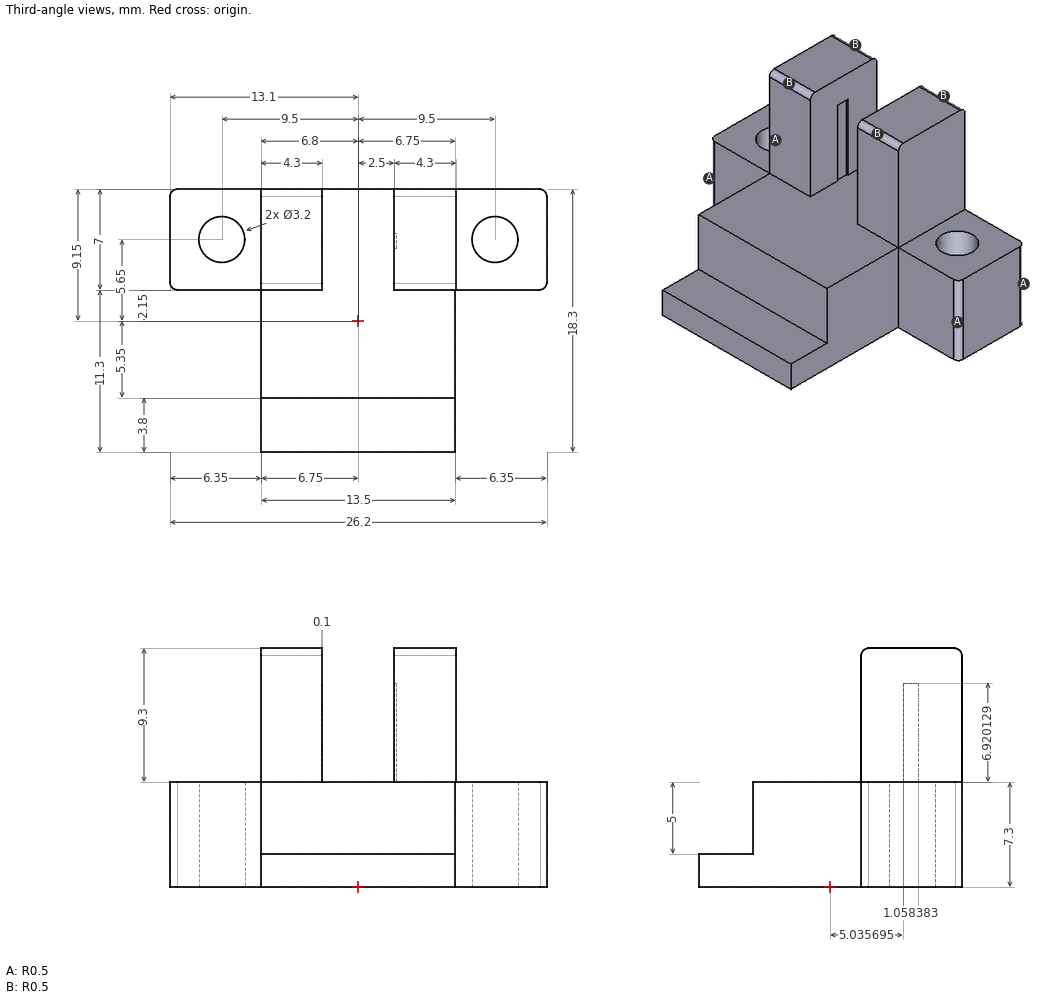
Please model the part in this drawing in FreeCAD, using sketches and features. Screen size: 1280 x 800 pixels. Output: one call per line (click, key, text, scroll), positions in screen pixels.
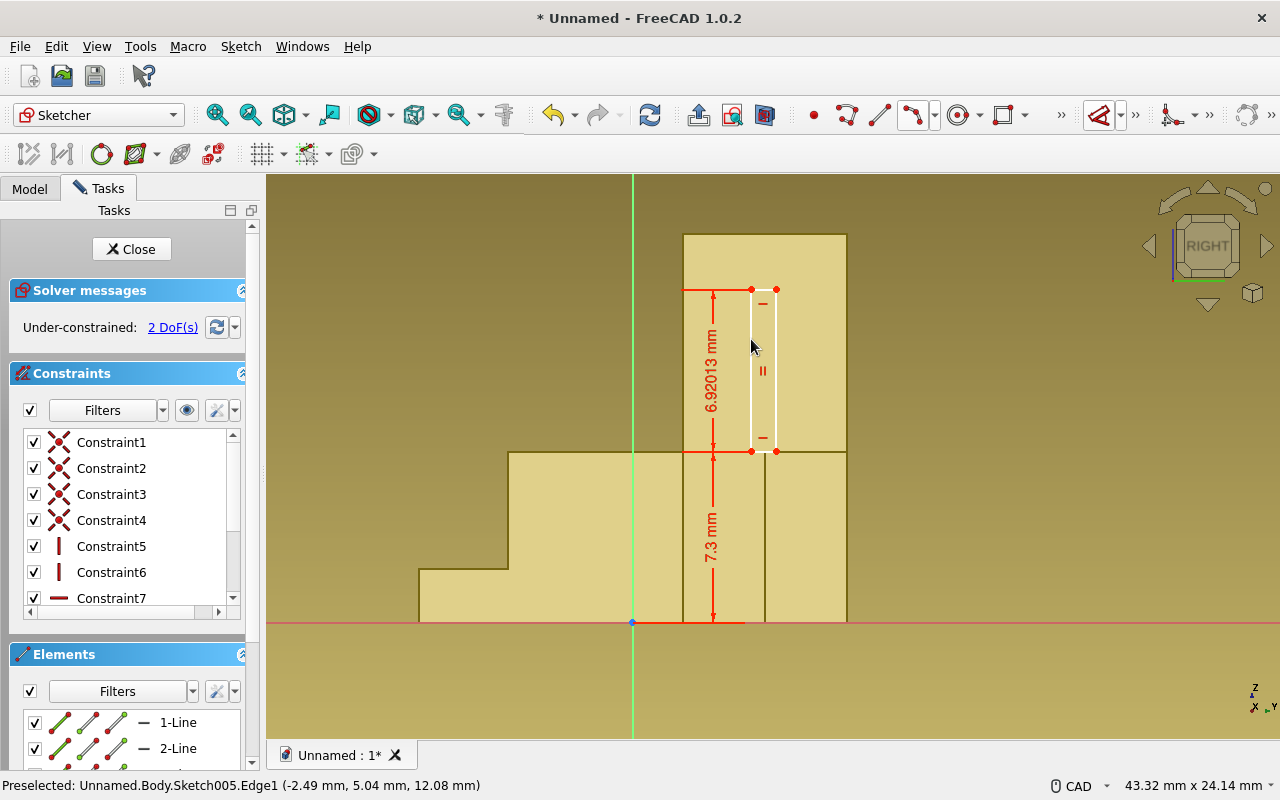
scroll(761, 452, up, 3)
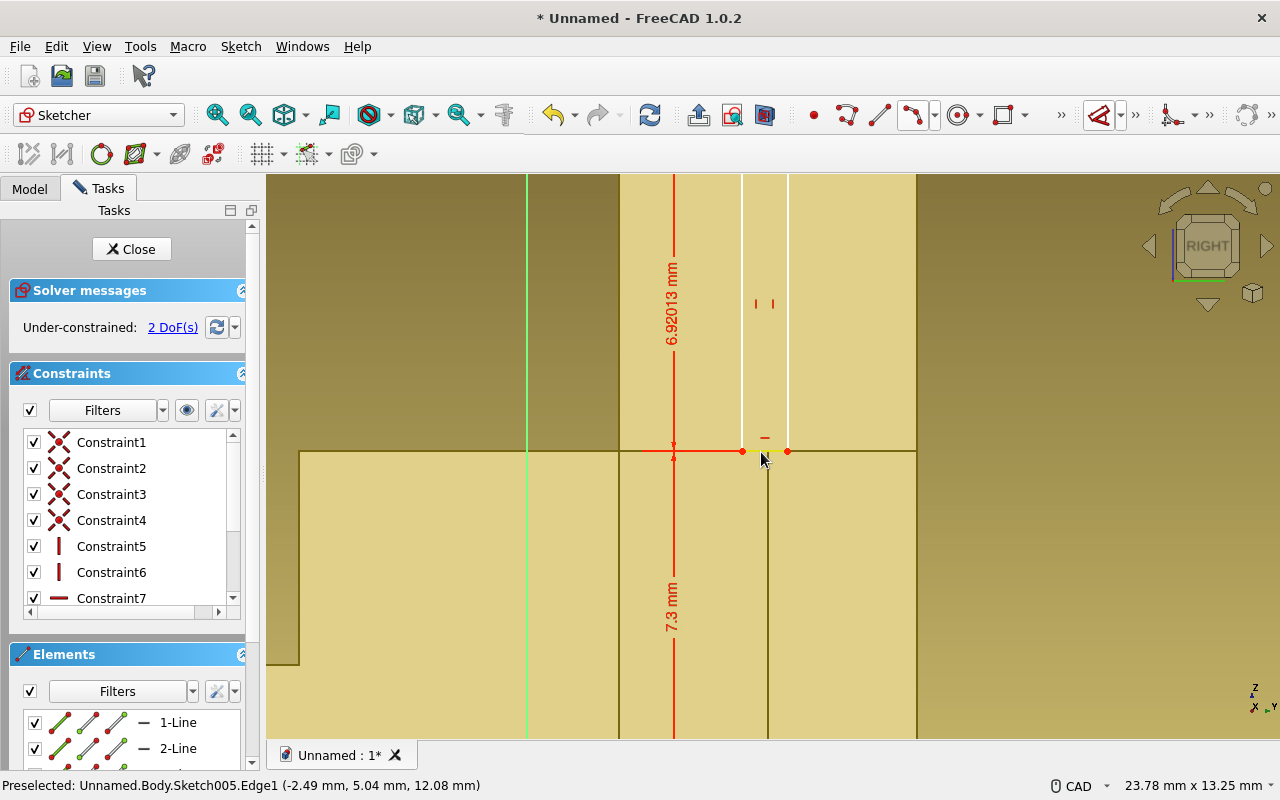
click(761, 451)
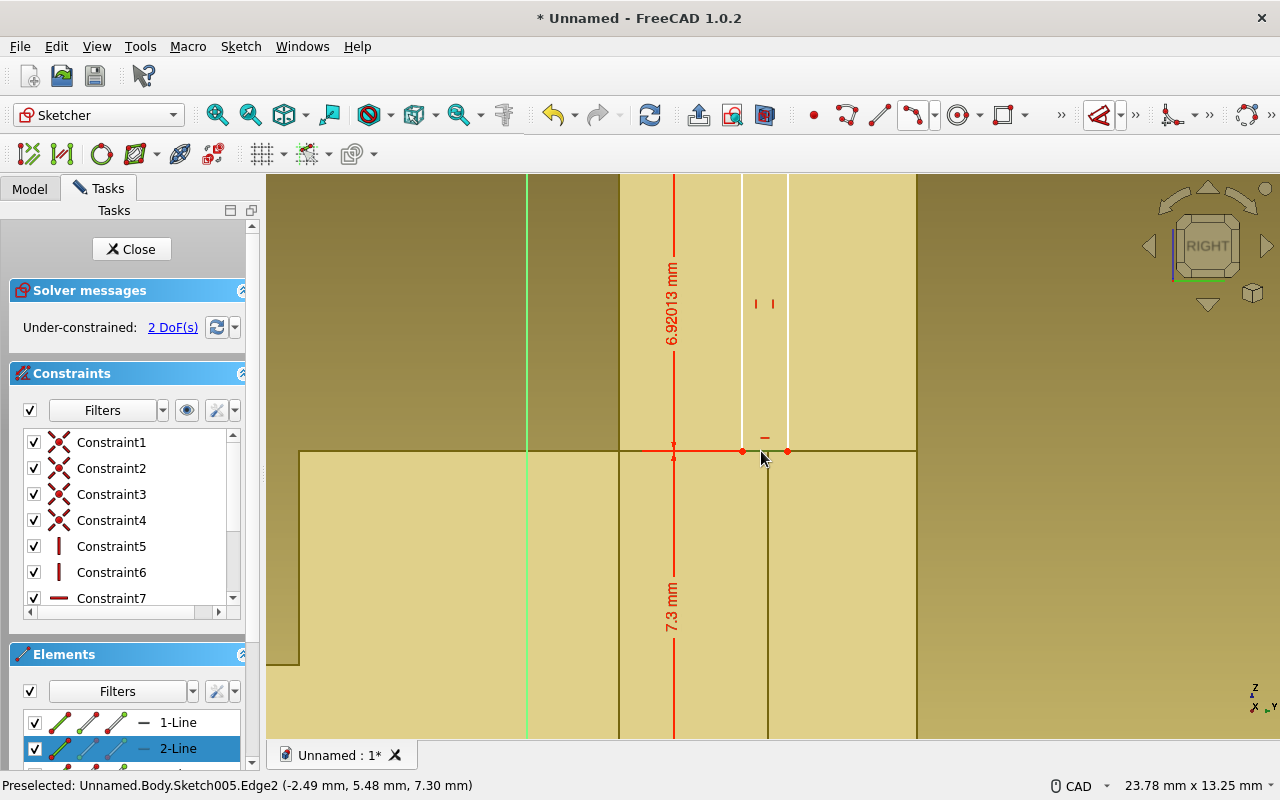
key(l)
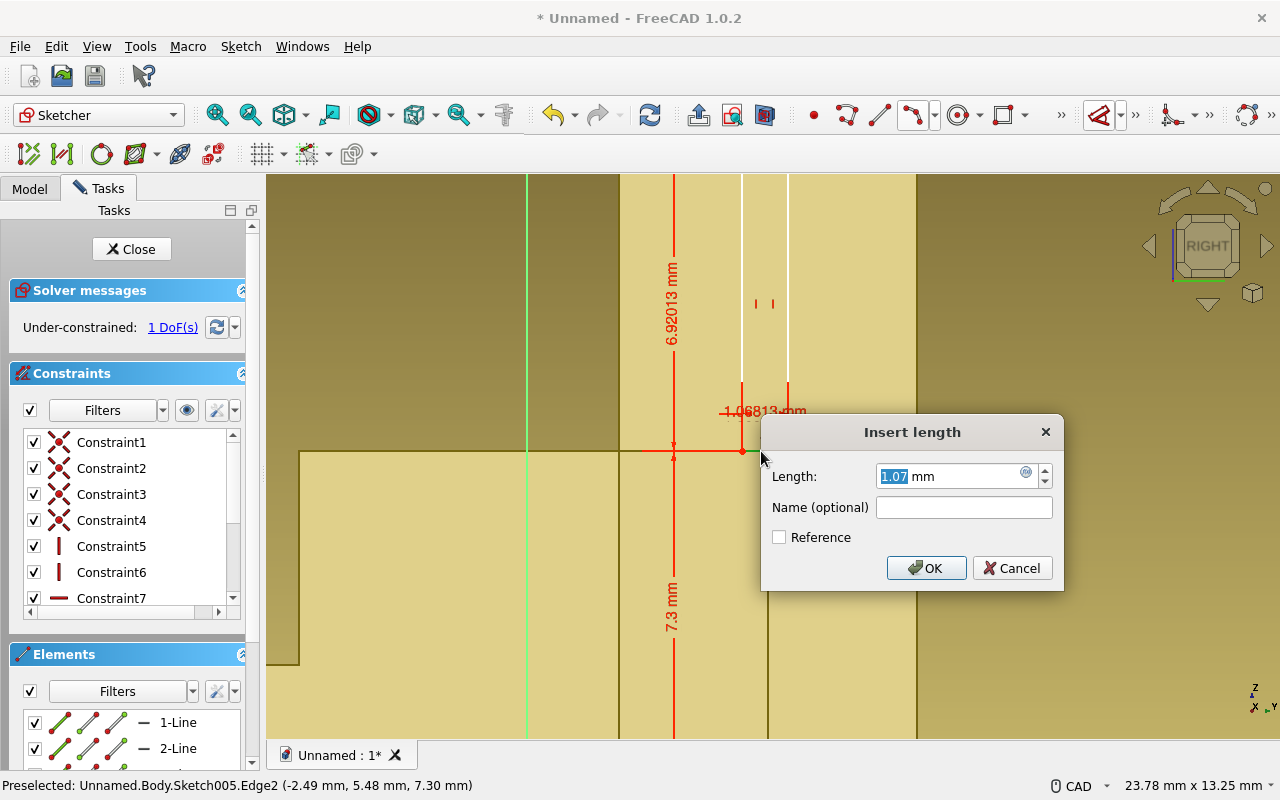
text(1.058383)
key(Return)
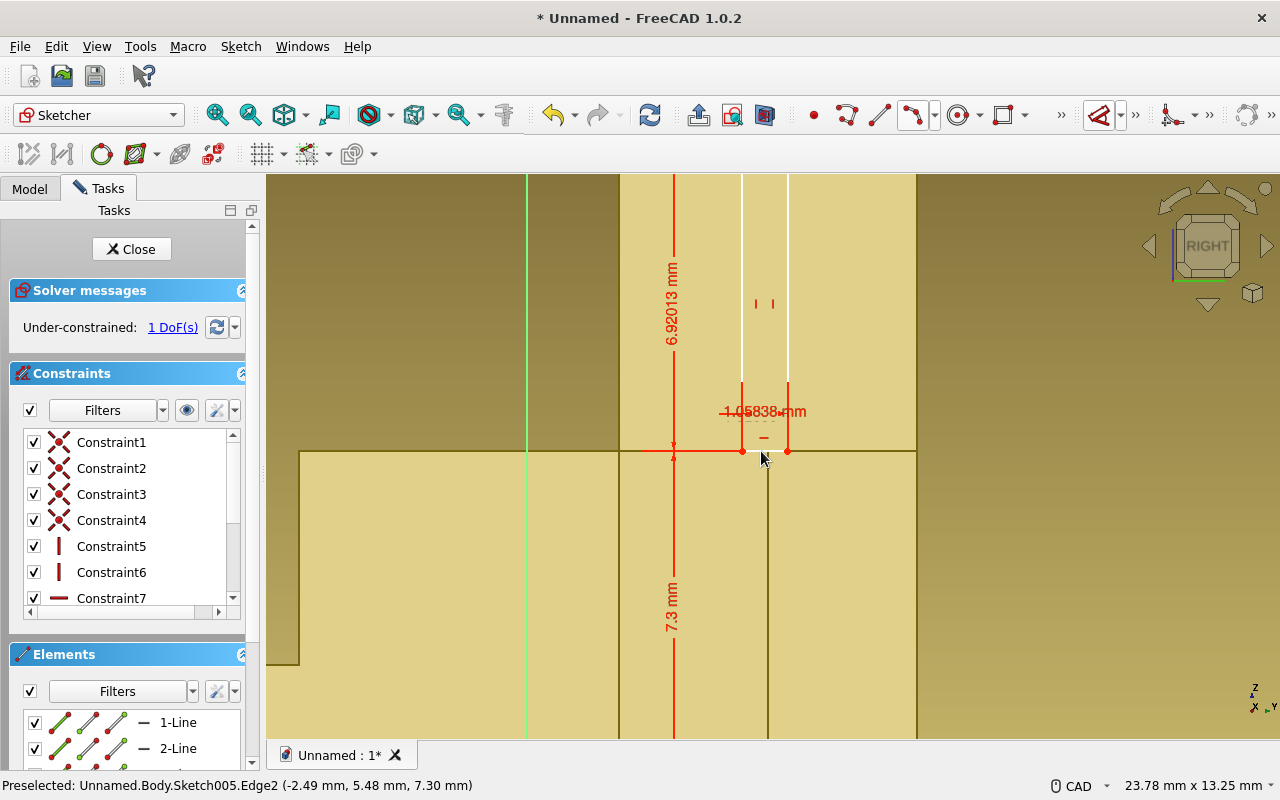
scroll(762, 453, down, 3)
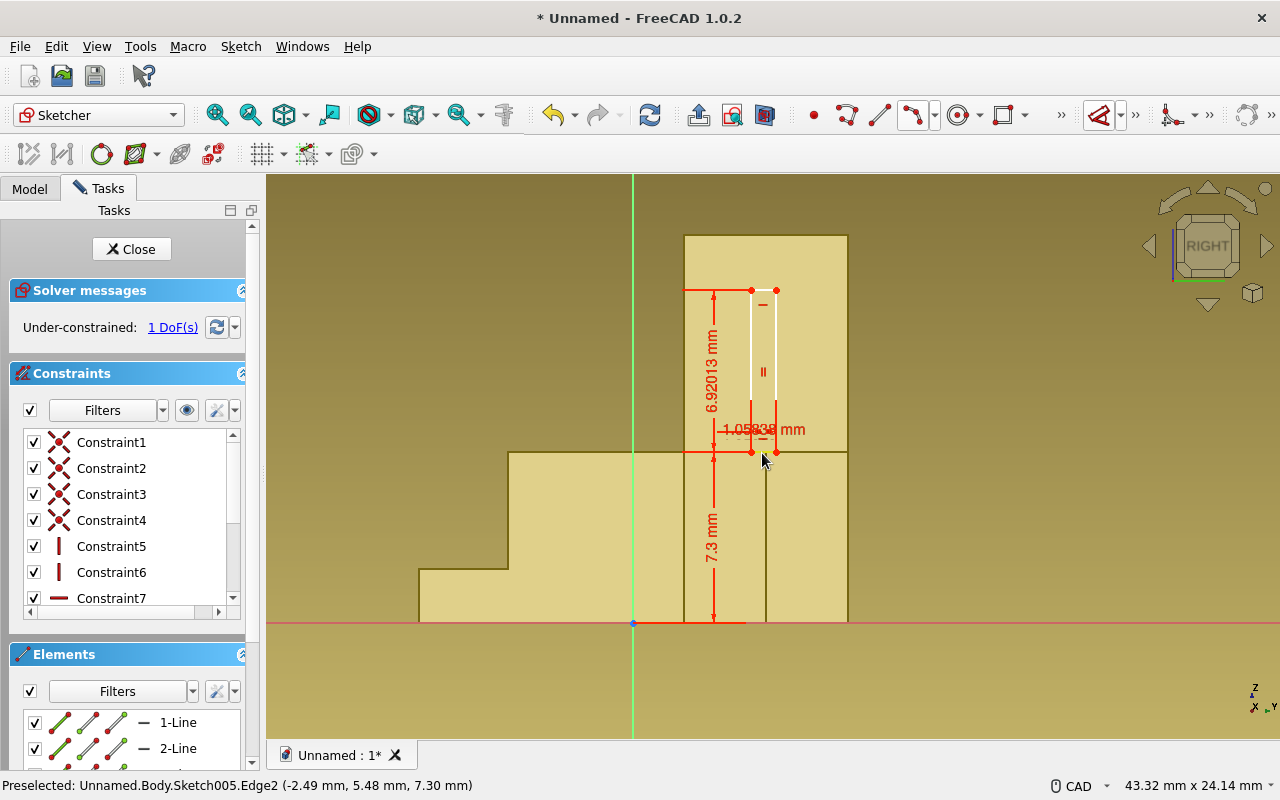
click(751, 290)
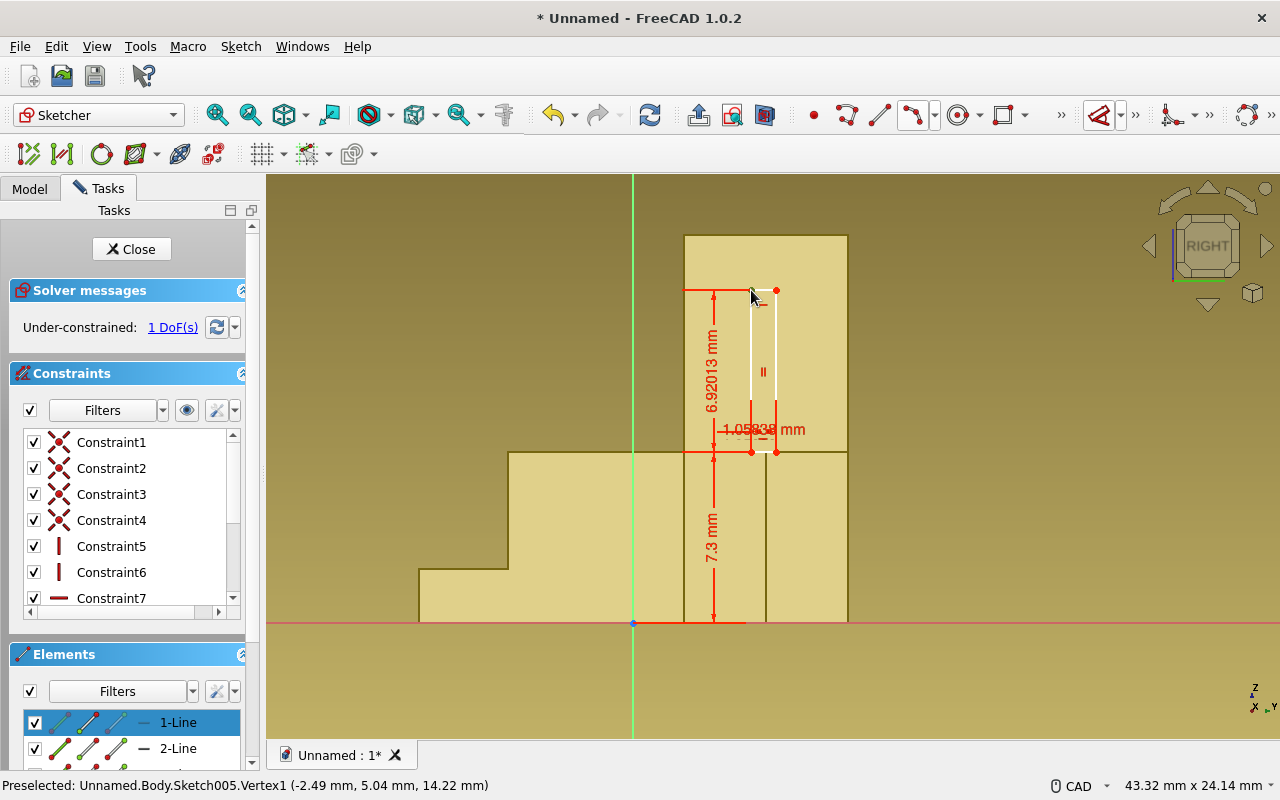
click(1120, 116)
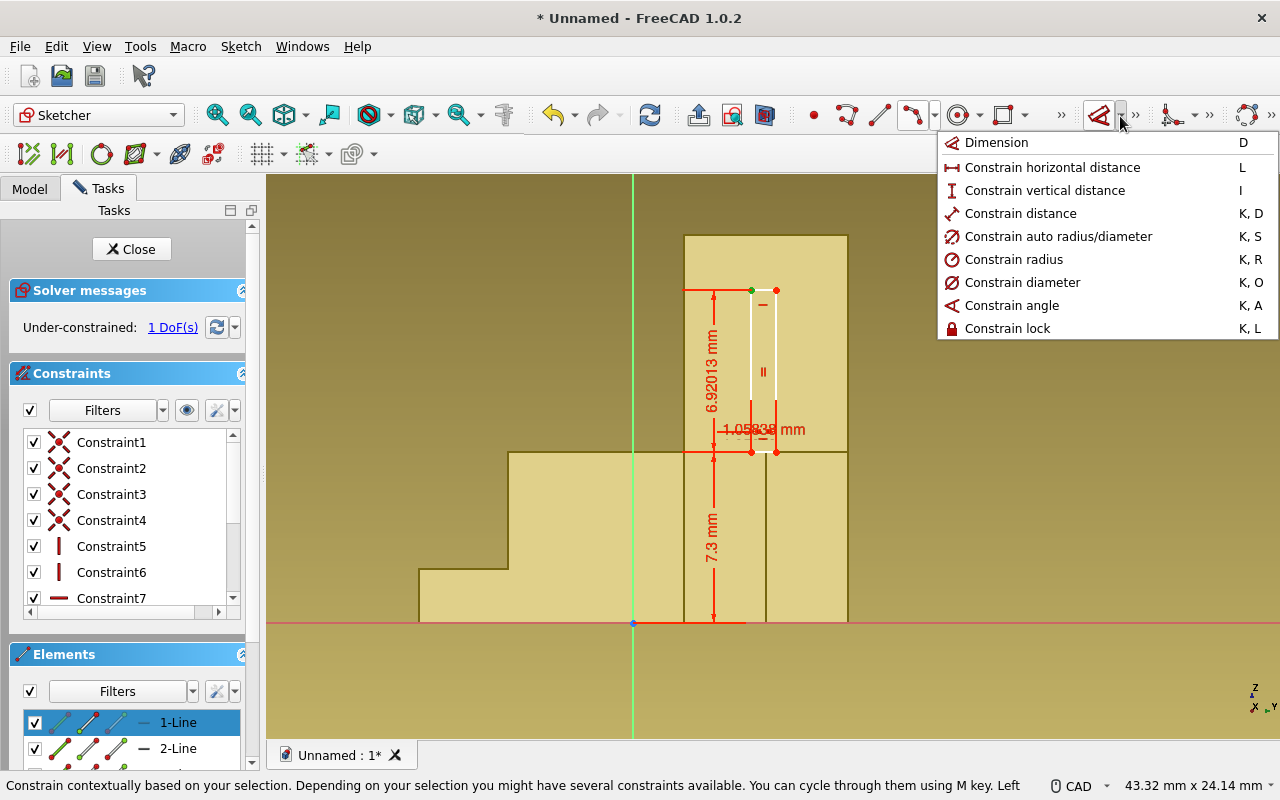
click(1108, 168)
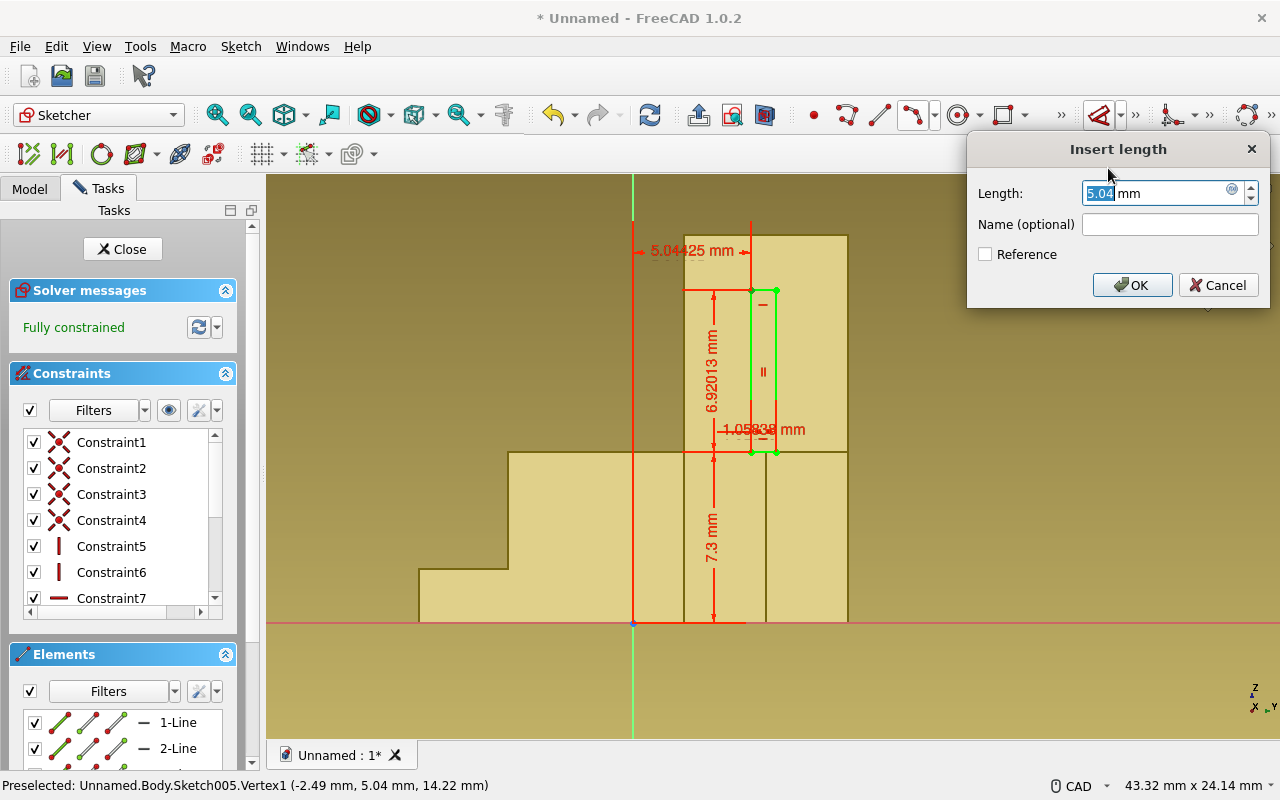
text(5.035695)
key(Return)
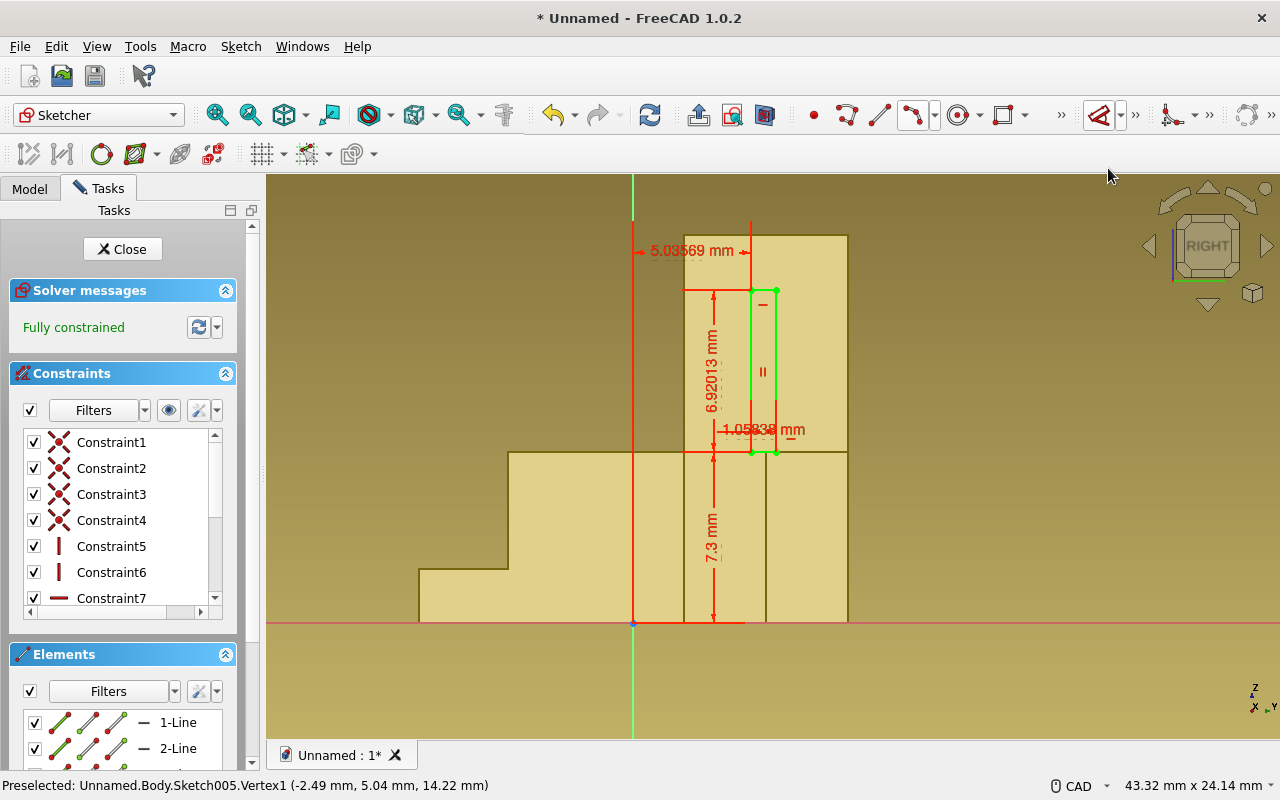
click(123, 249)